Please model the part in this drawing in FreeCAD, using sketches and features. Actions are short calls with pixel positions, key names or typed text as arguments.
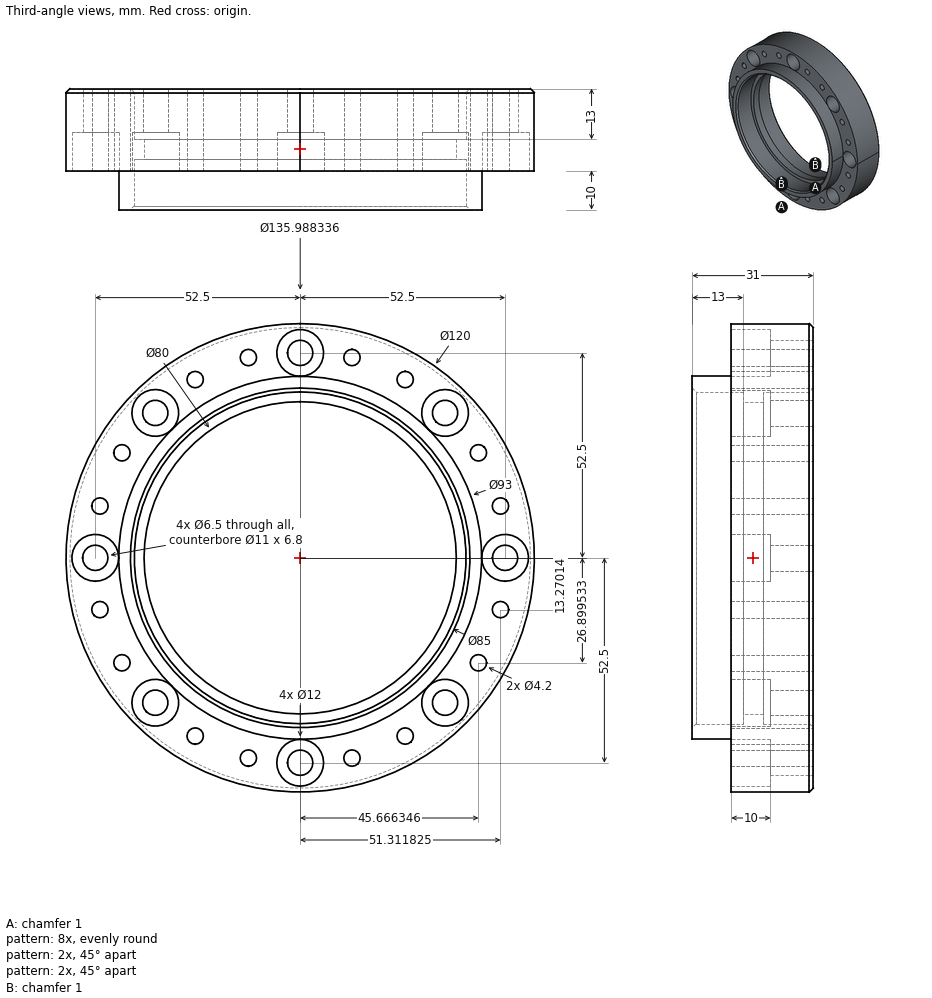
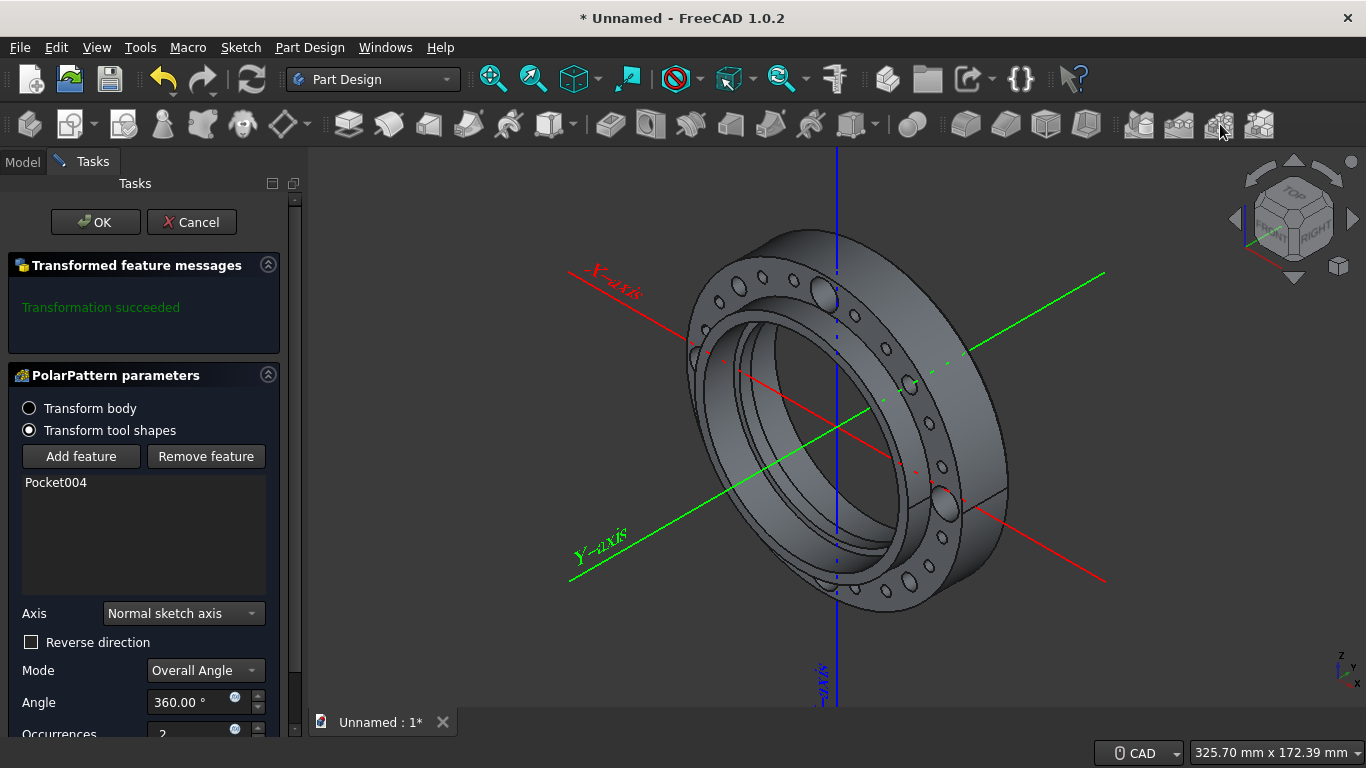
click(184, 614)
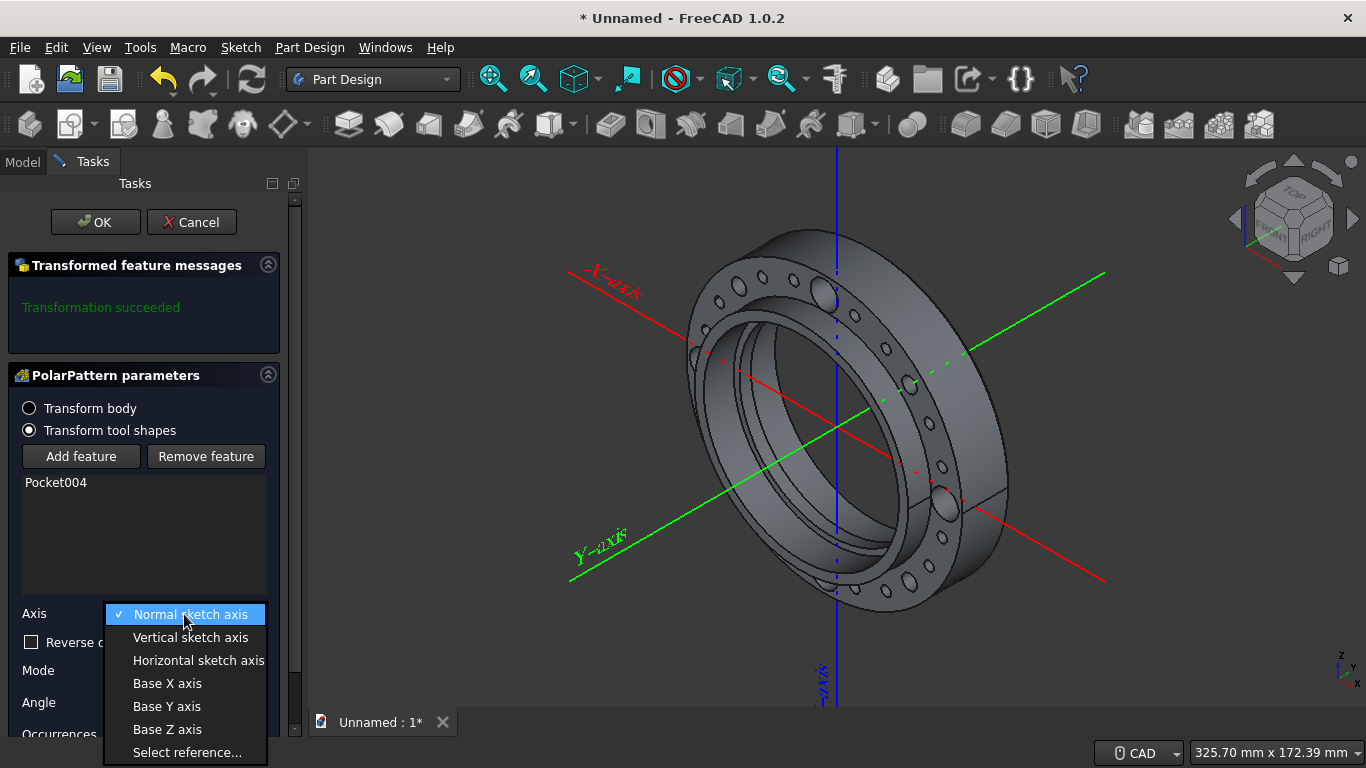
click(184, 706)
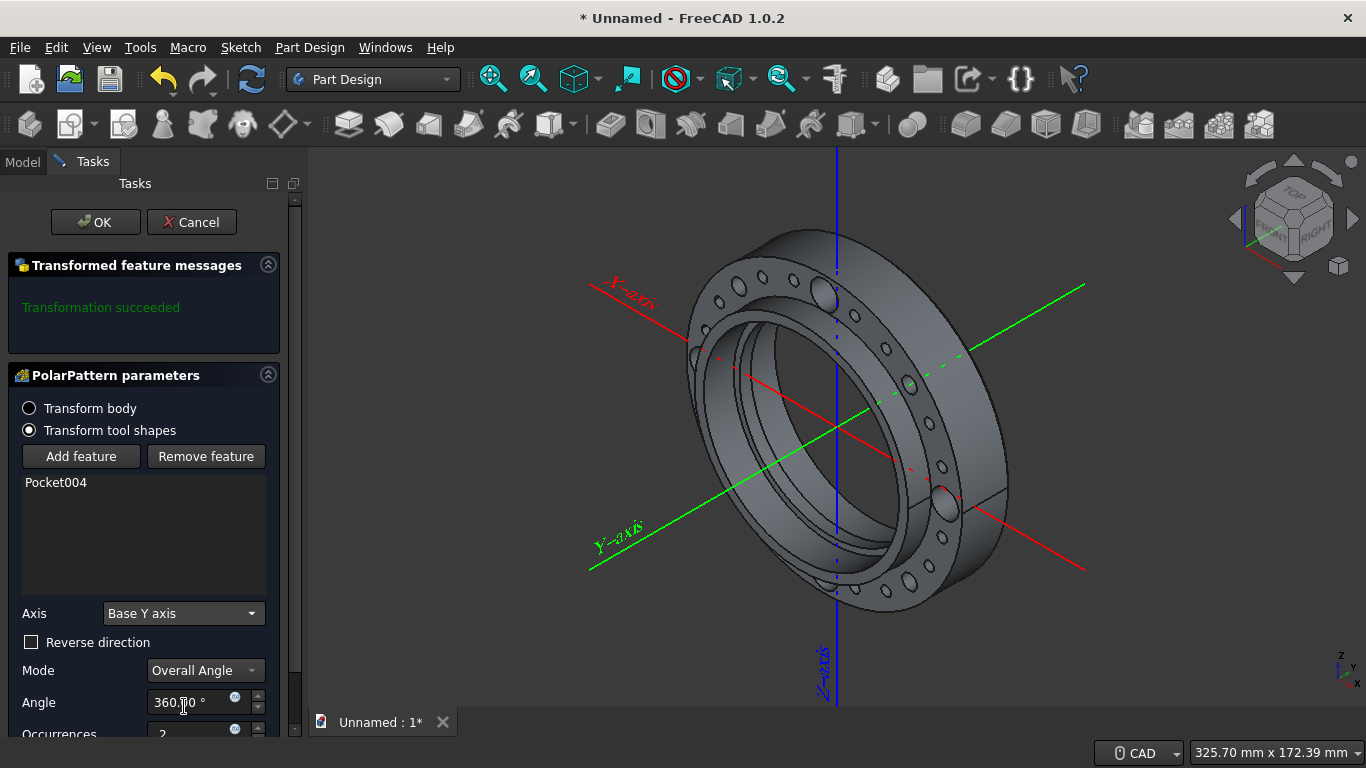
click(206, 670)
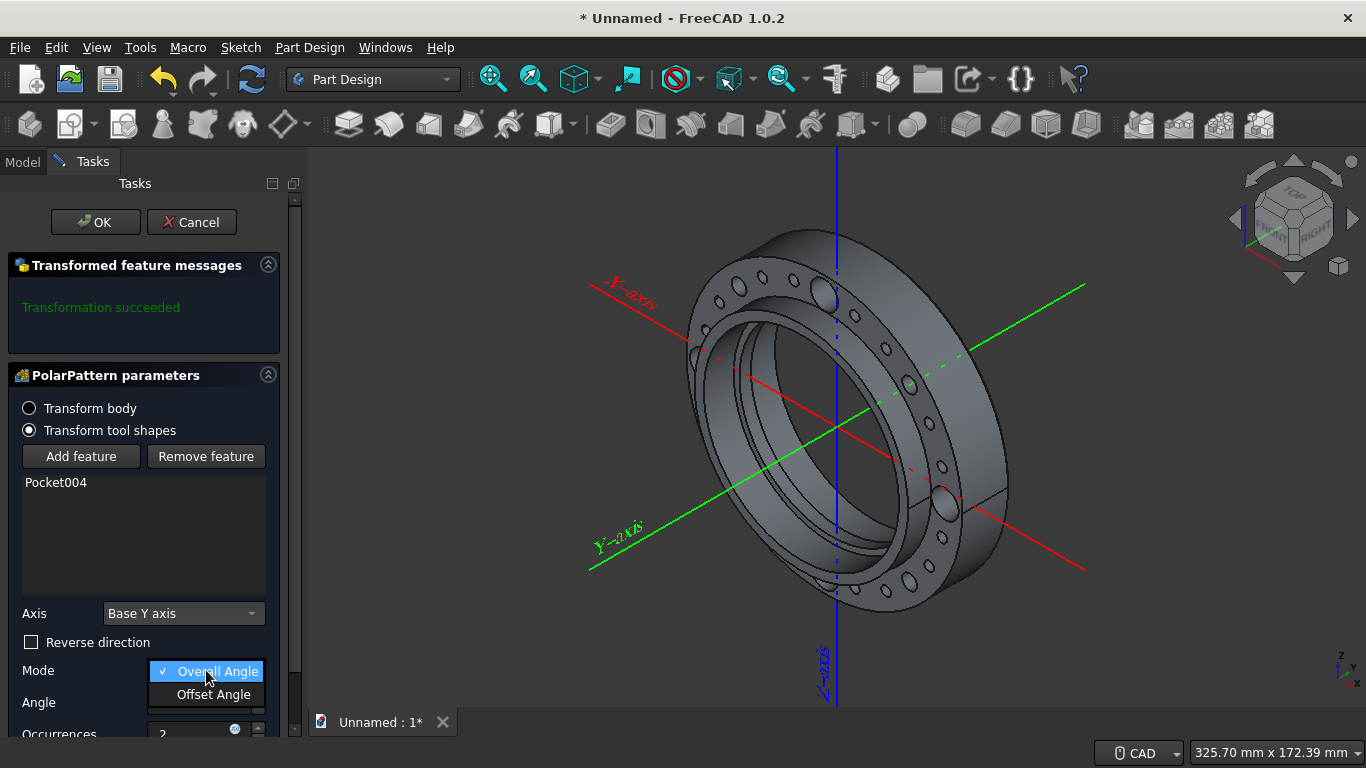
click(206, 694)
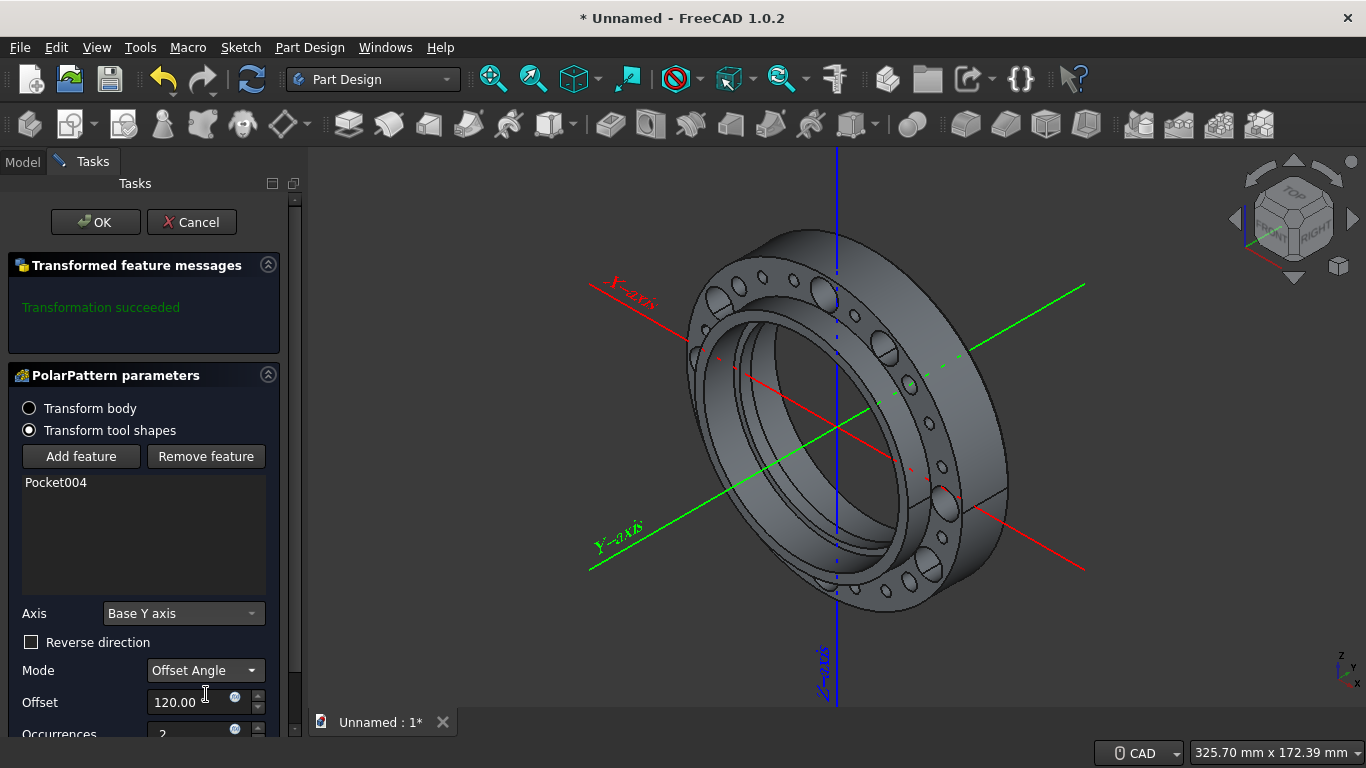
triple_click(198, 702)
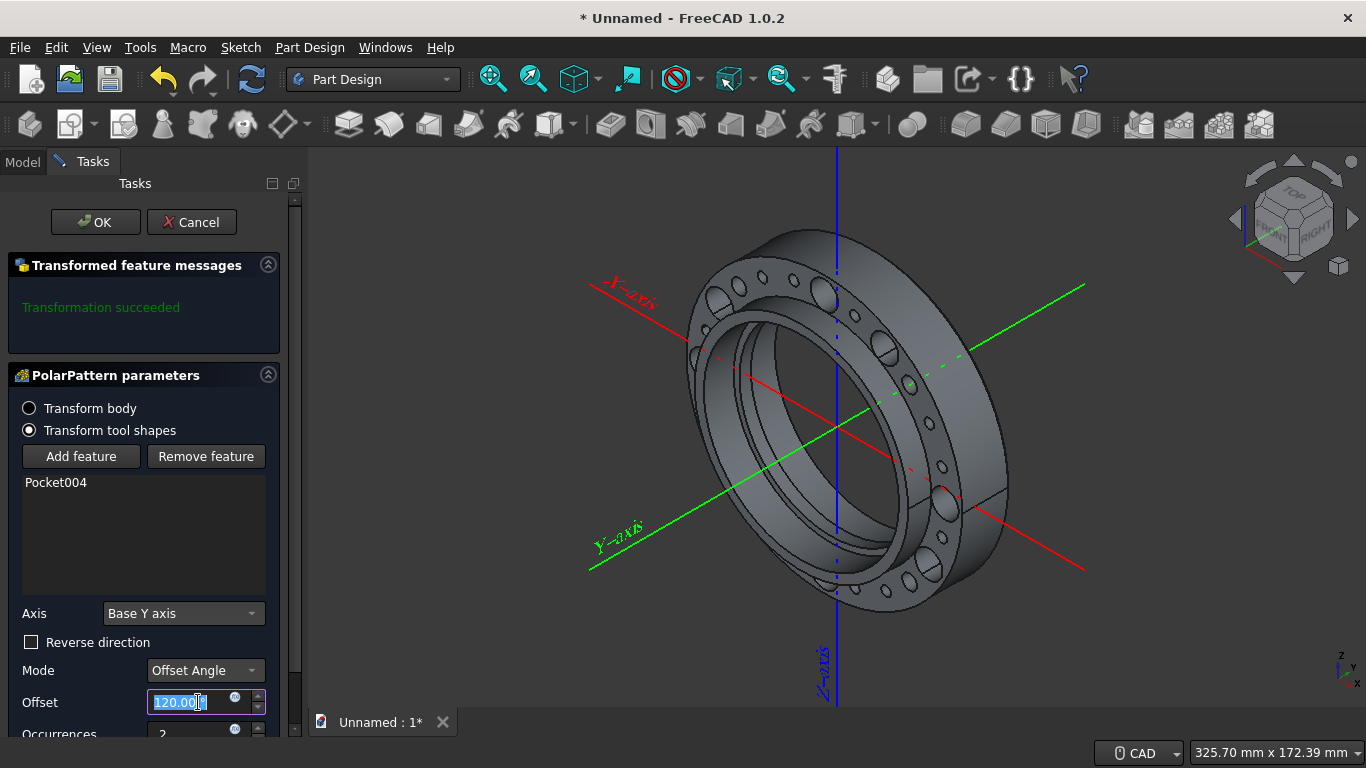
text(45)
key(Tab)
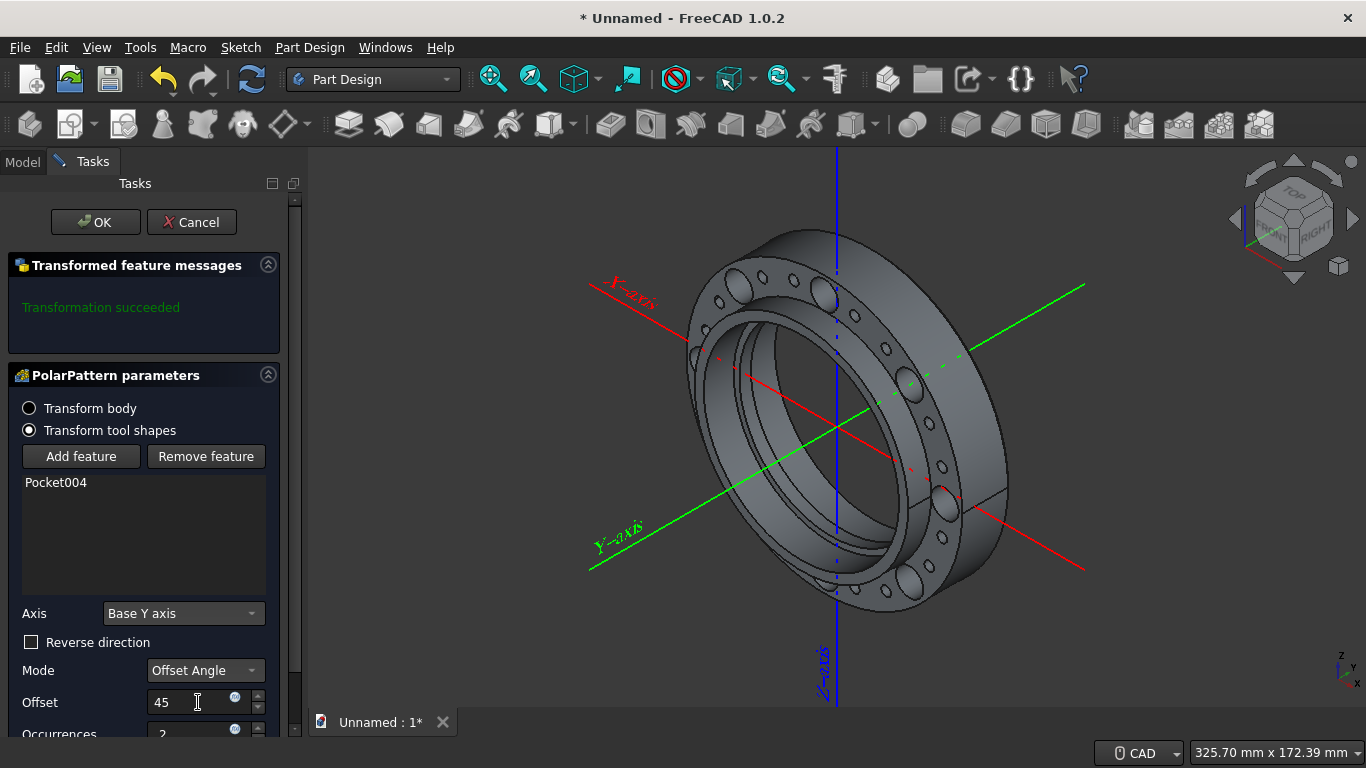
scroll(295, 464, down, 2)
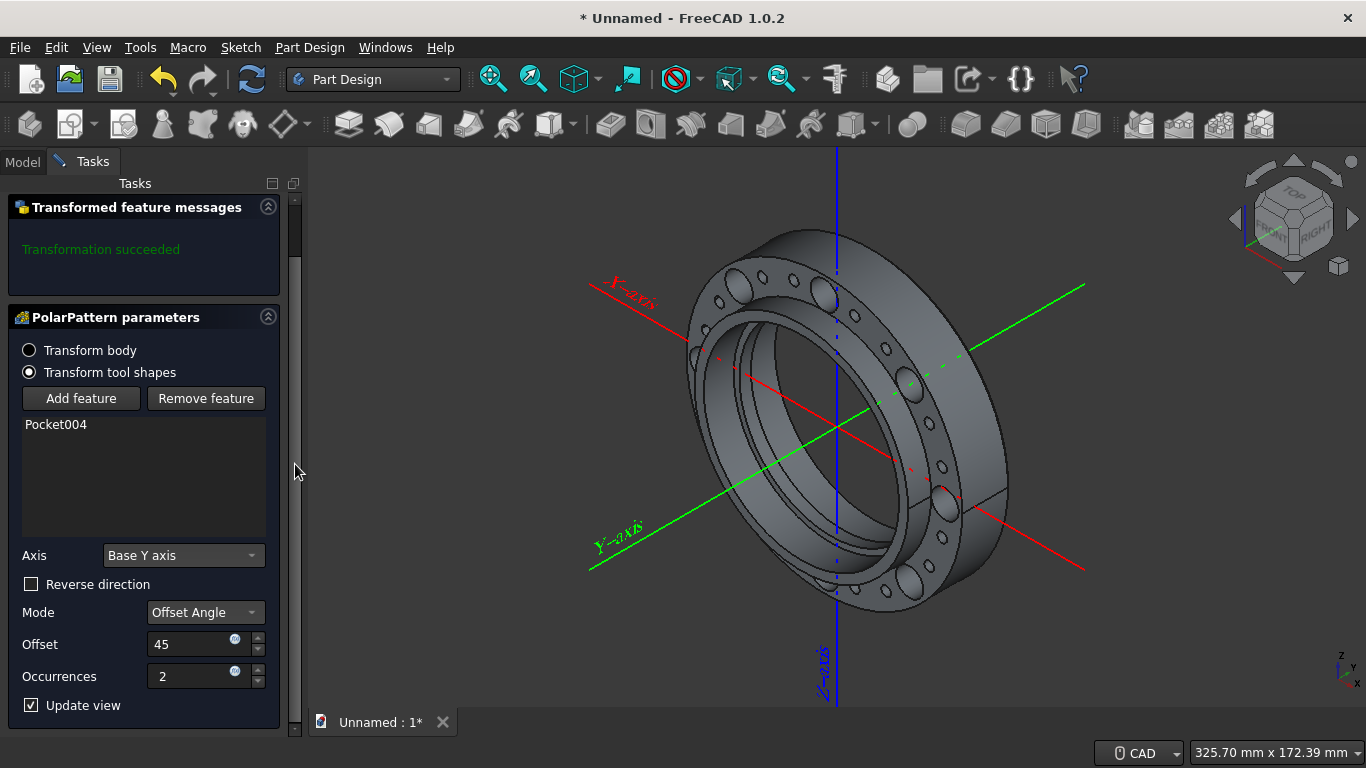
triple_click(198, 676)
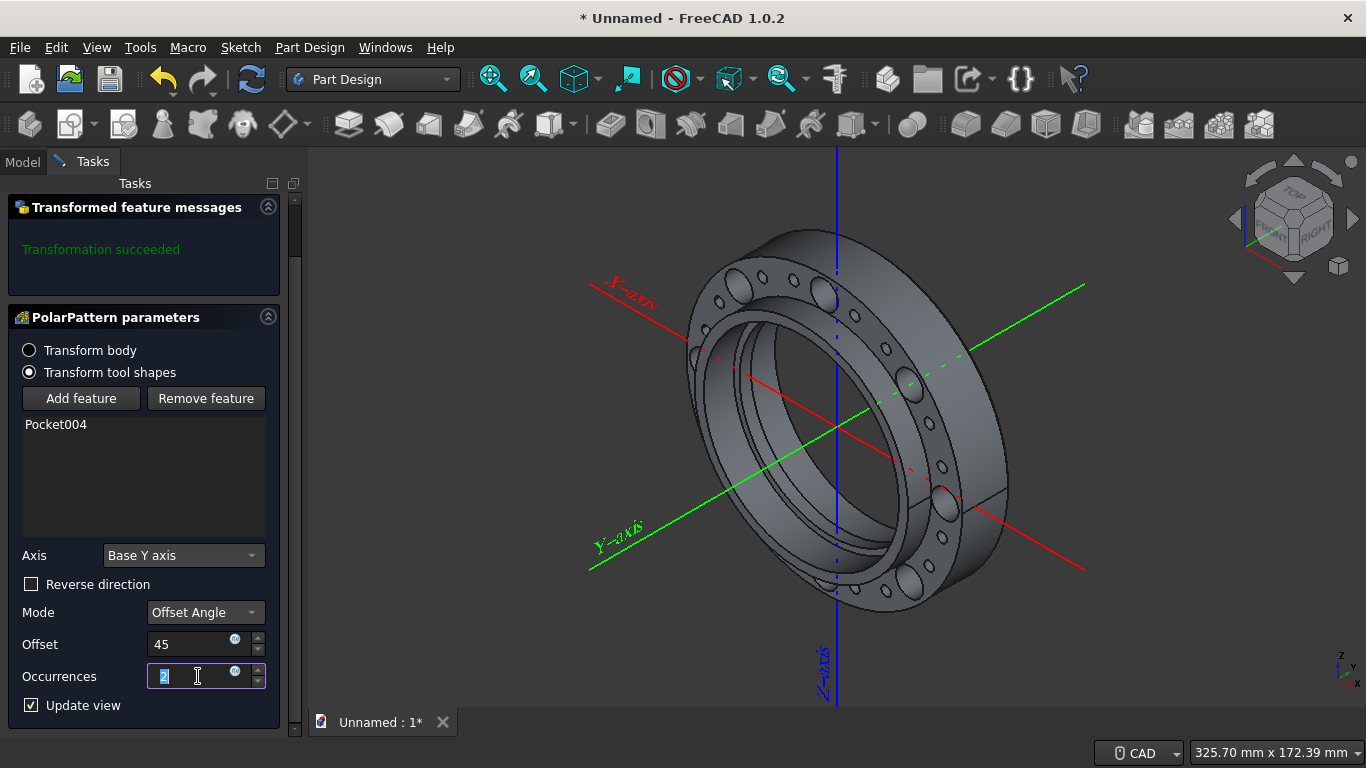
text(2)
key(Tab)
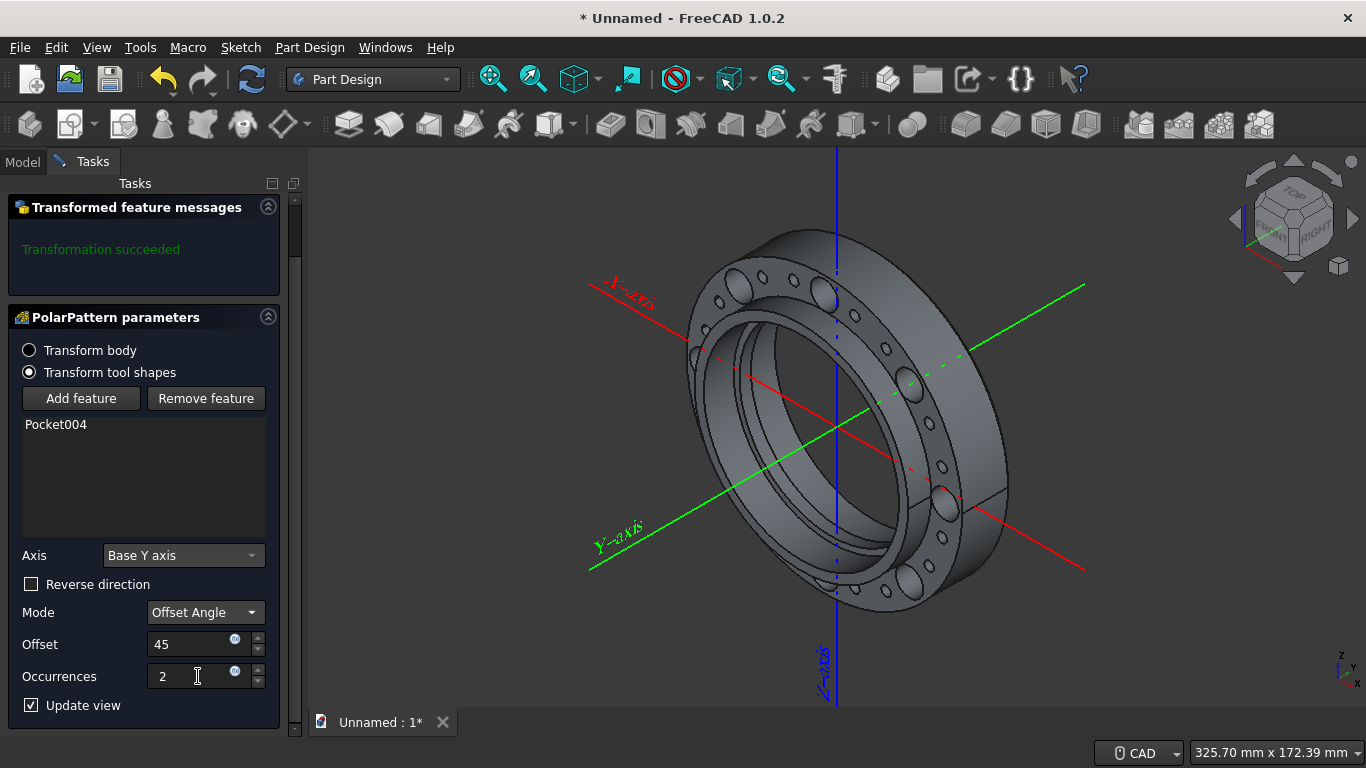
scroll(295, 464, up, 2)